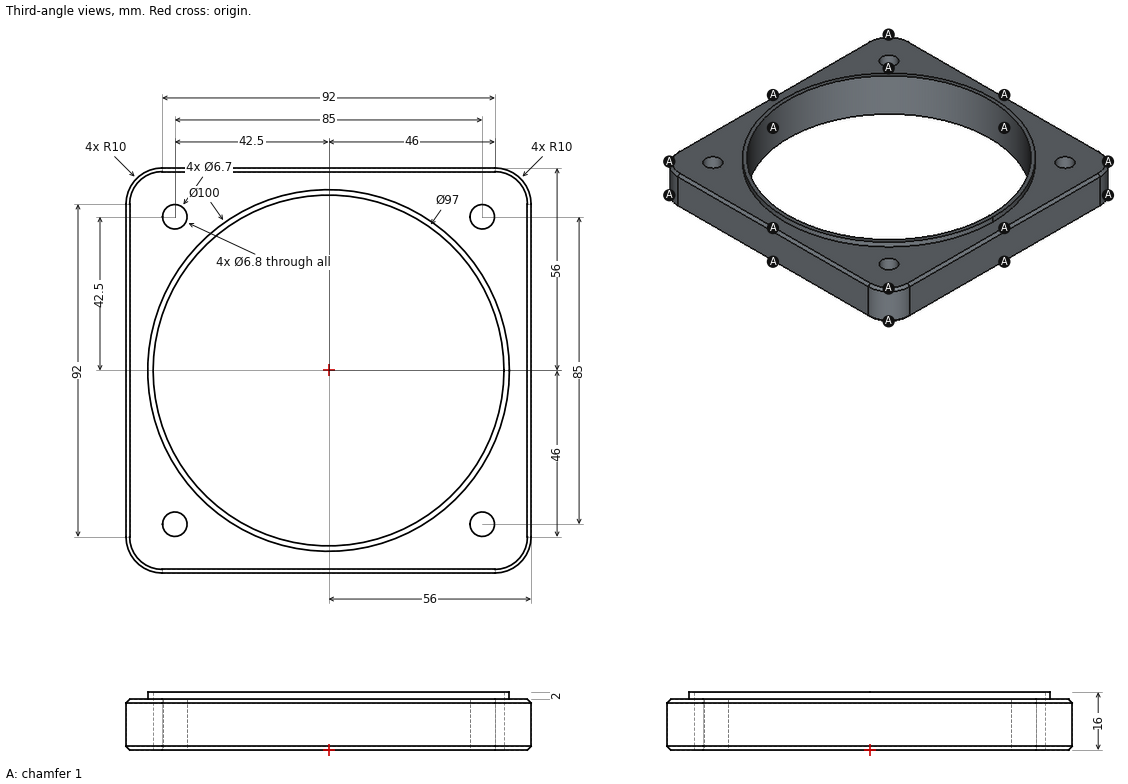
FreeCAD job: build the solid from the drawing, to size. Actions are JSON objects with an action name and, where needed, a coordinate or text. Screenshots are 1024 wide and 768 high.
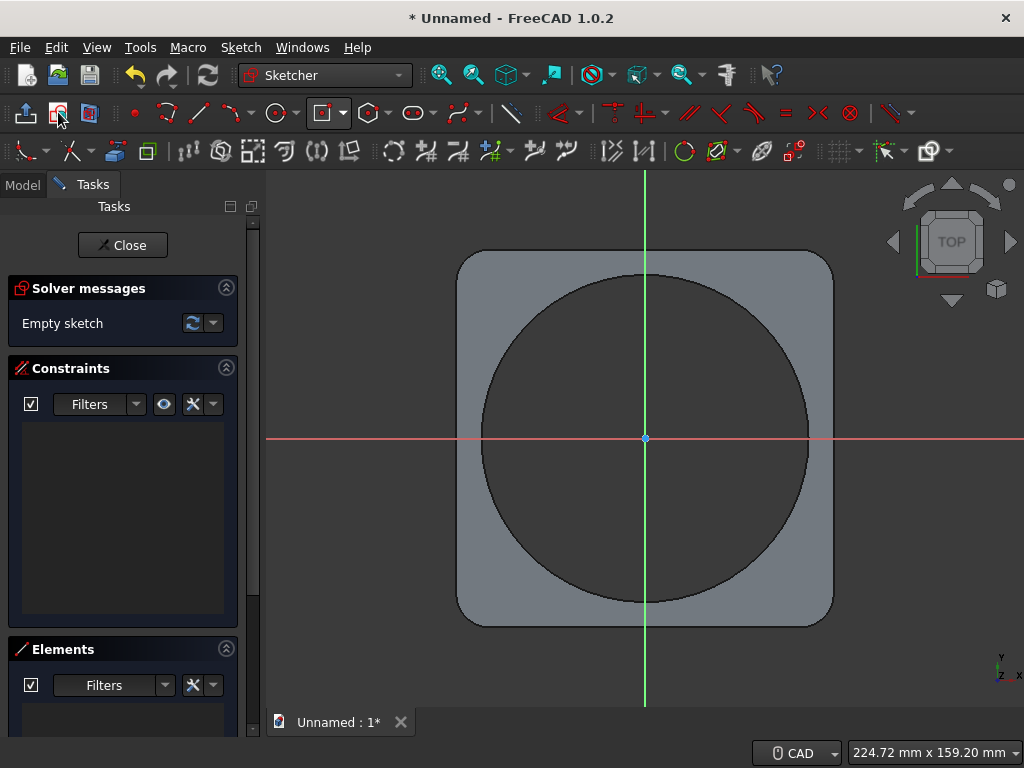
{"action": "left_click", "coordinate": [276, 114]}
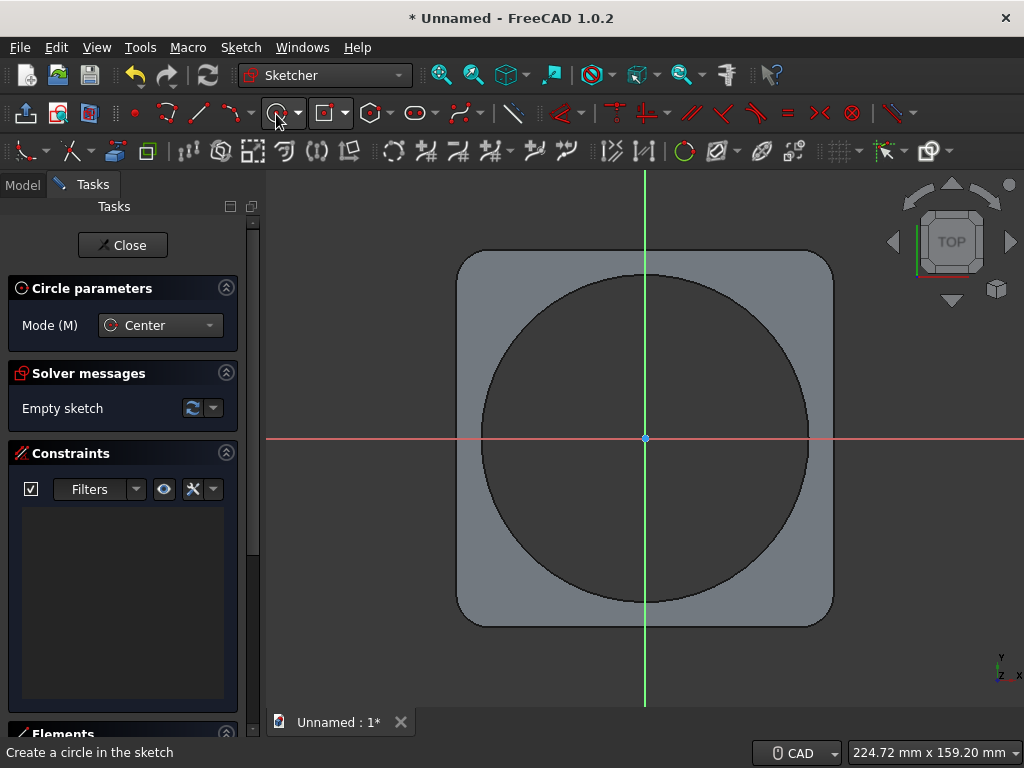
{"action": "scroll", "coordinate": [502, 295], "scroll_direction": "up", "scroll_amount": 4}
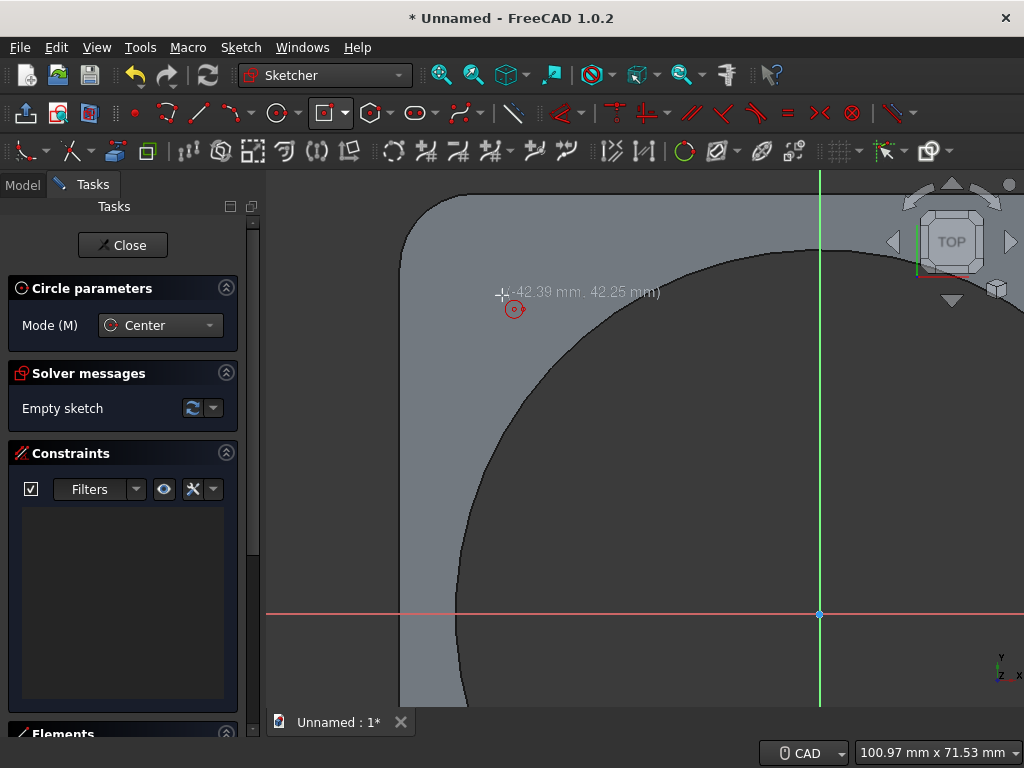
{"action": "left_click", "coordinate": [501, 295]}
{"action": "mouse_move", "coordinate": [519, 277]}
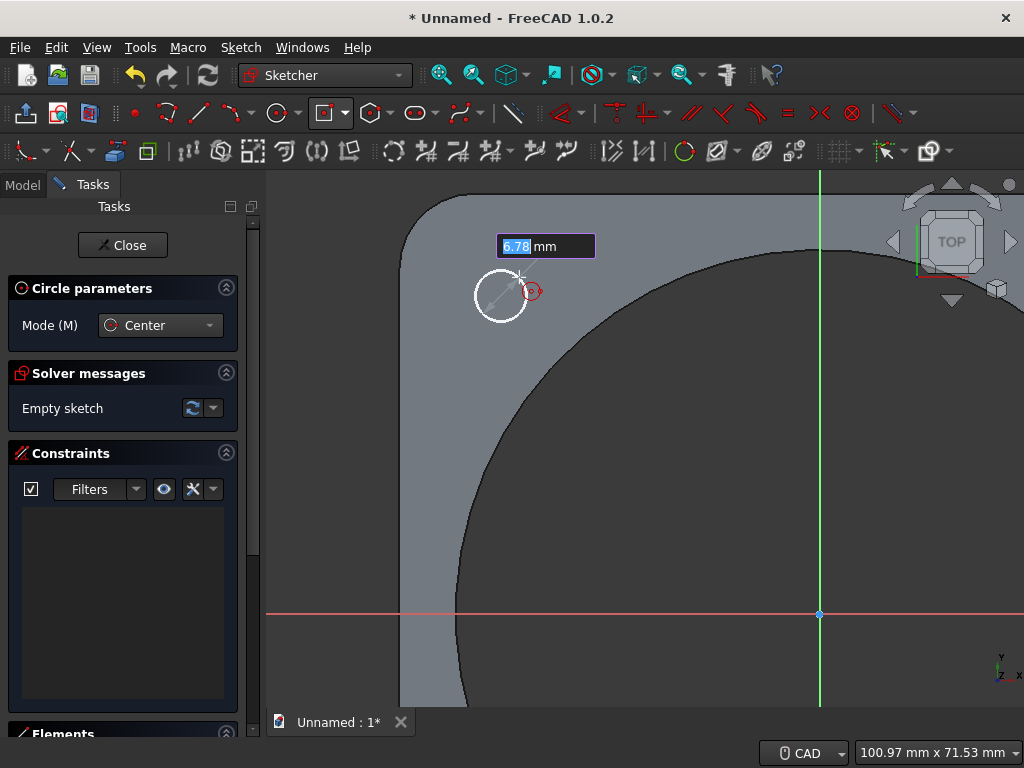
{"action": "type", "text": "6.7"}
{"action": "key", "text": "Return"}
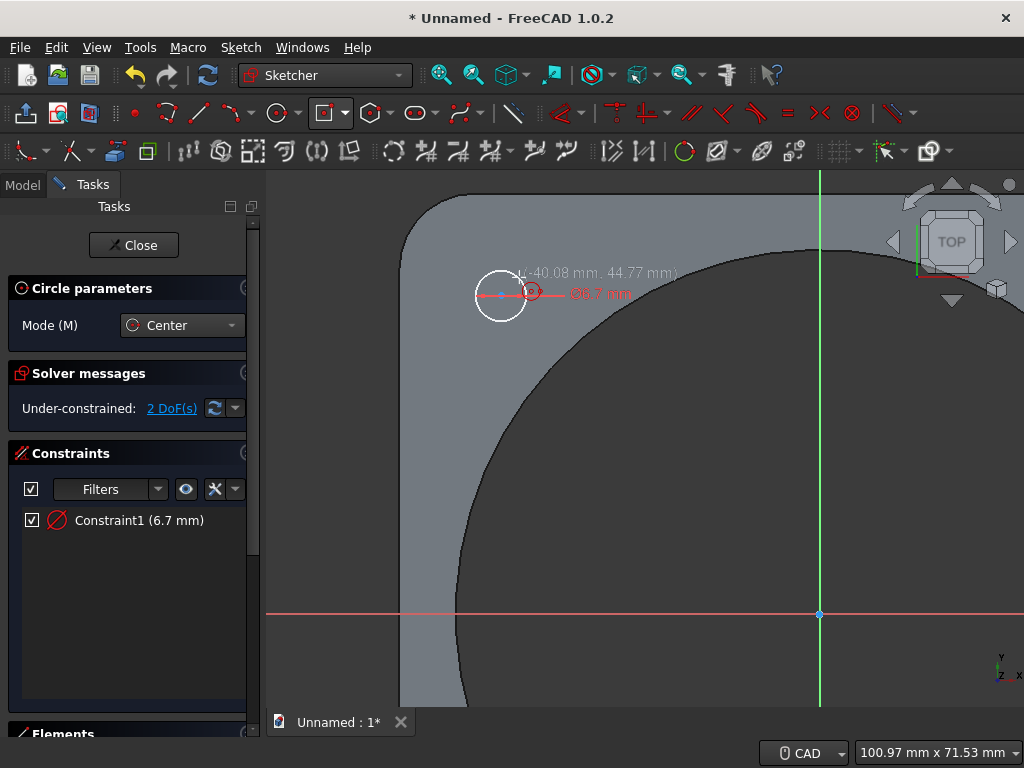
{"action": "scroll", "coordinate": [378, 295], "scroll_direction": "down", "scroll_amount": 4}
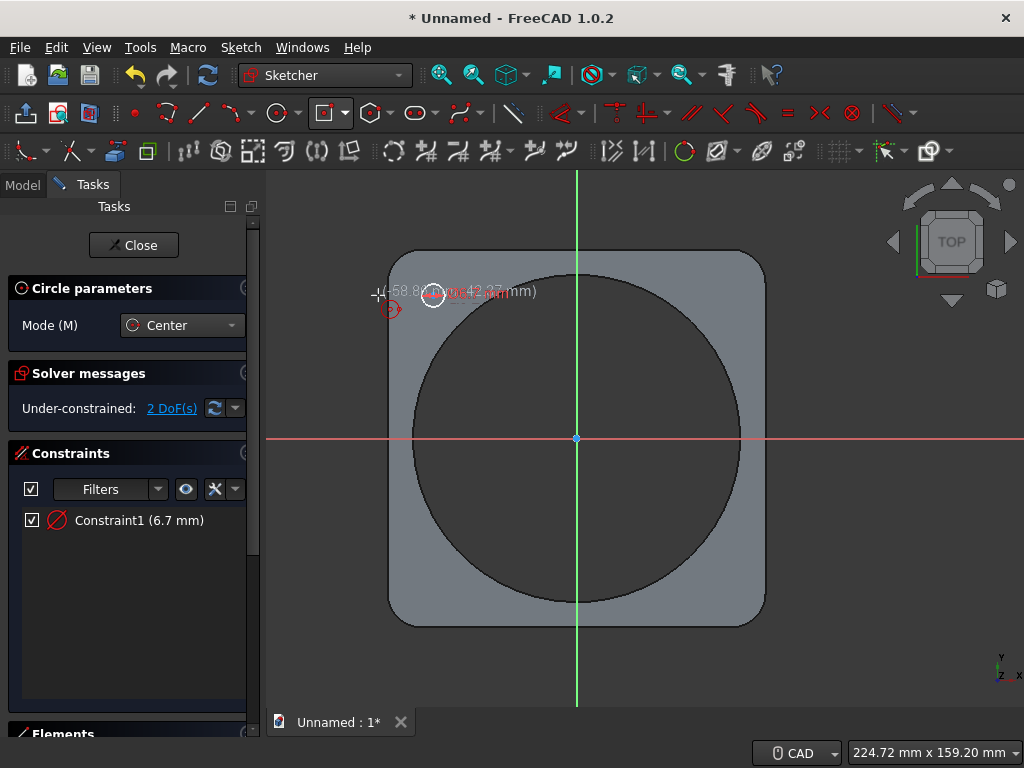
{"action": "scroll", "coordinate": [720, 295], "scroll_direction": "up", "scroll_amount": 4}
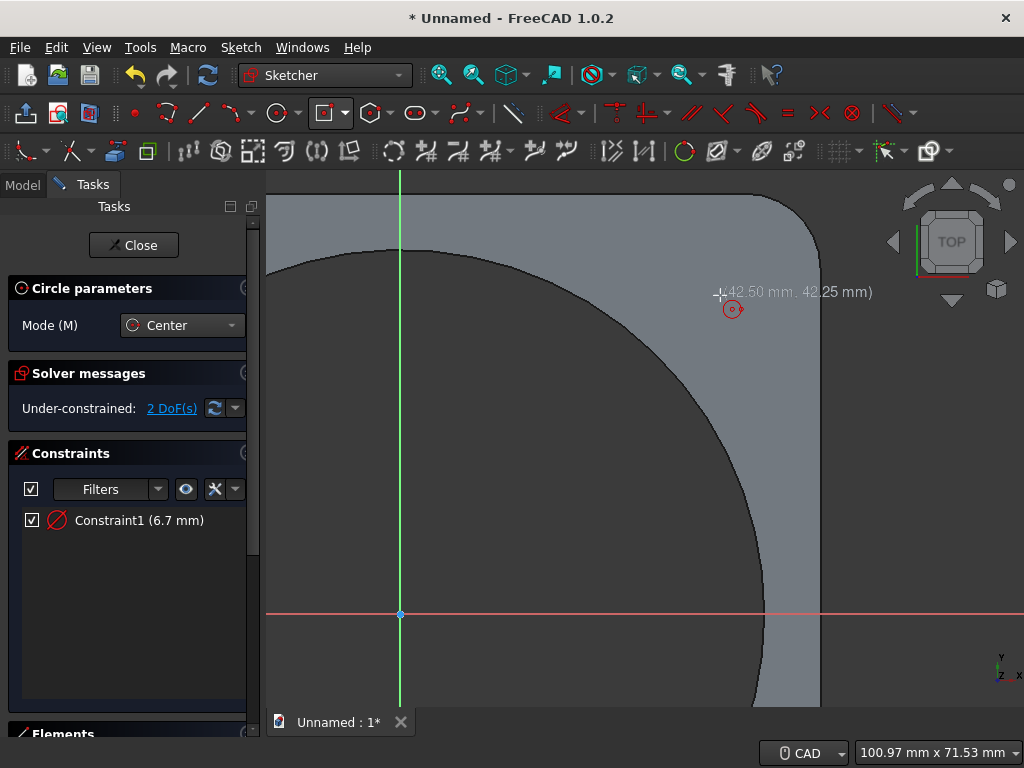
{"action": "left_click", "coordinate": [719, 295]}
{"action": "mouse_move", "coordinate": [737, 277]}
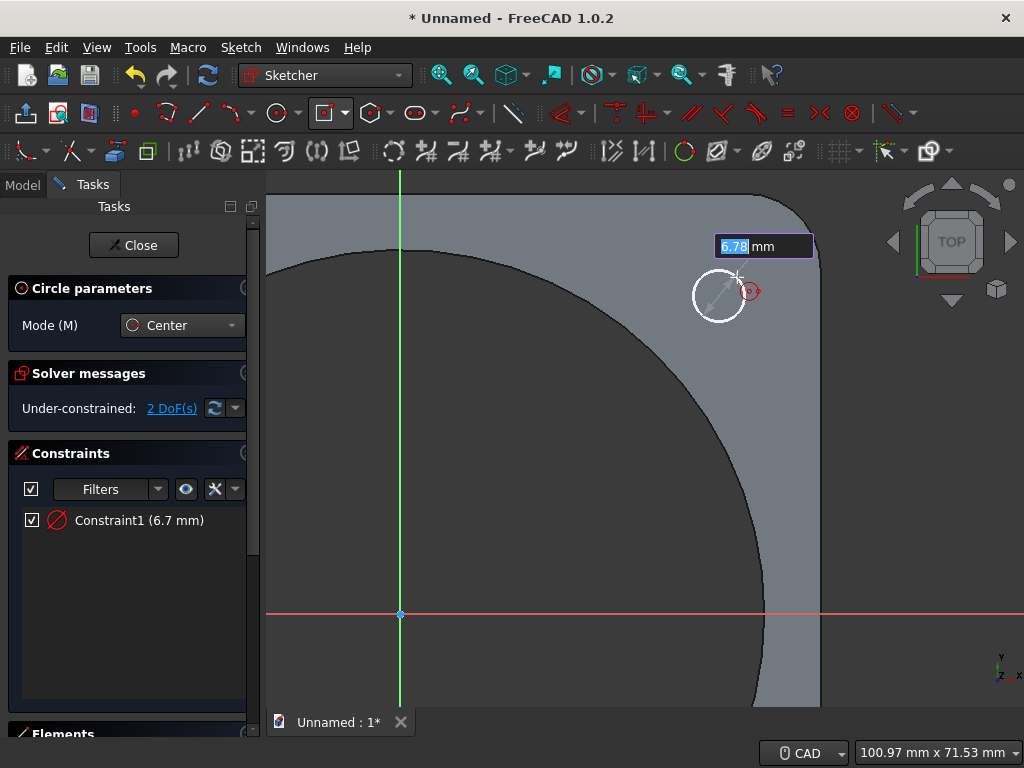
{"action": "type", "text": "6.7"}
{"action": "key", "text": "Return"}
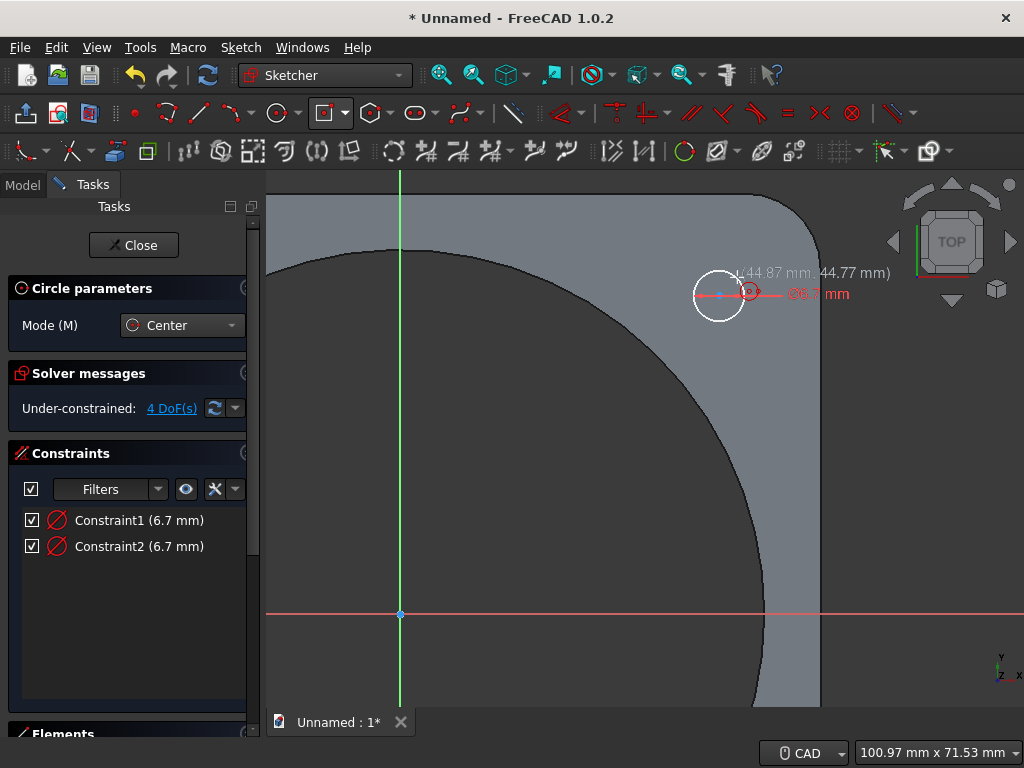
{"action": "scroll", "coordinate": [720, 295], "scroll_direction": "down", "scroll_amount": 4}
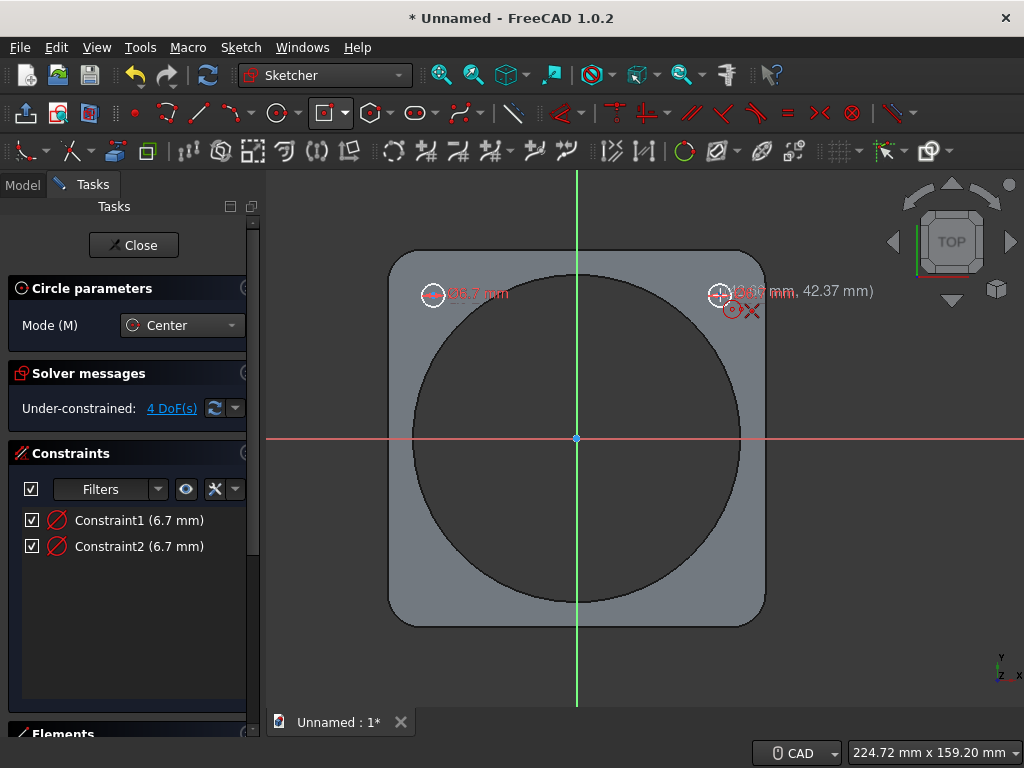
{"action": "scroll", "coordinate": [720, 582], "scroll_direction": "up", "scroll_amount": 4}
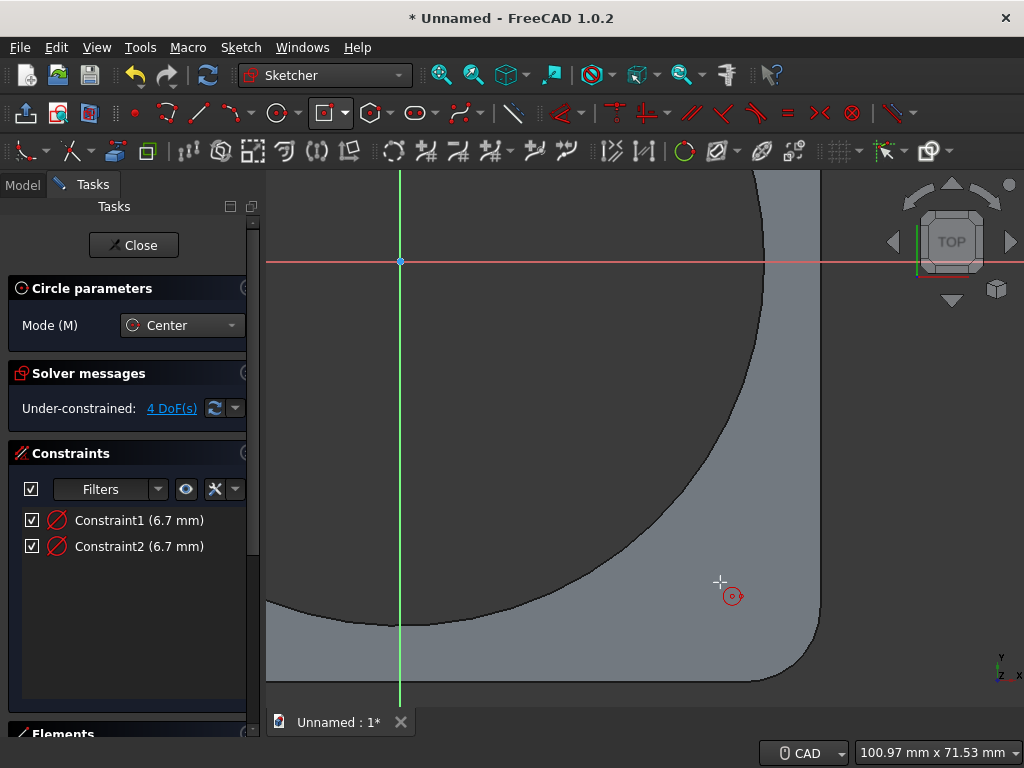
{"action": "left_click", "coordinate": [719, 581]}
{"action": "mouse_move", "coordinate": [737, 563]}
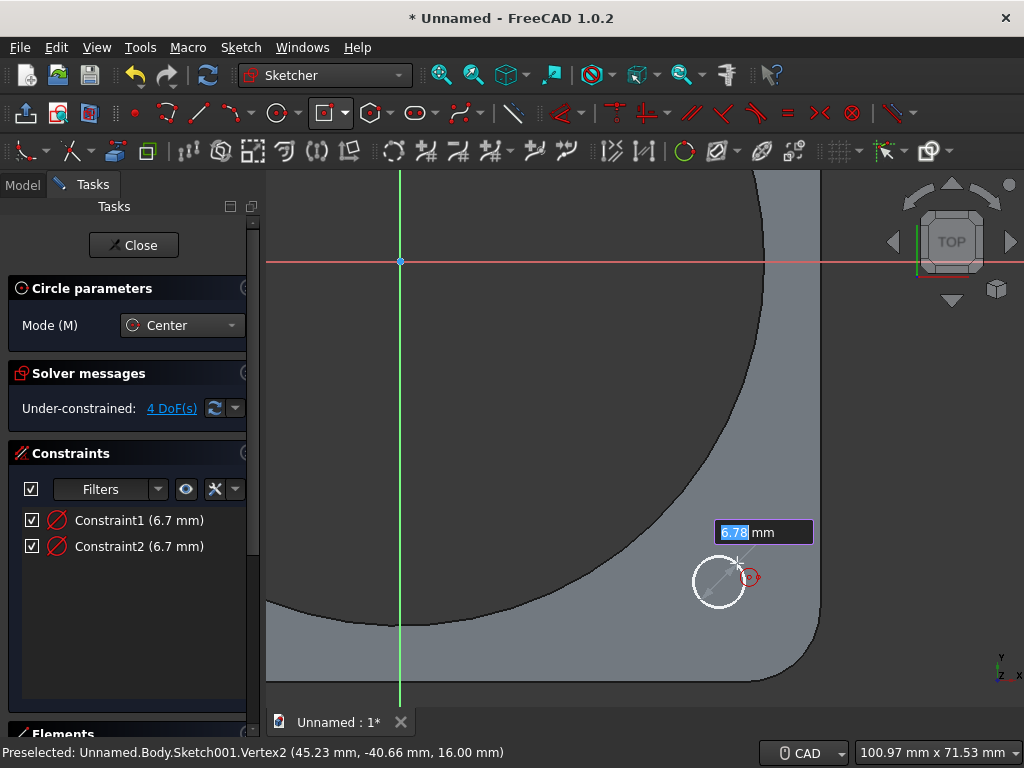
{"action": "type", "text": "6.7"}
{"action": "key", "text": "Return"}